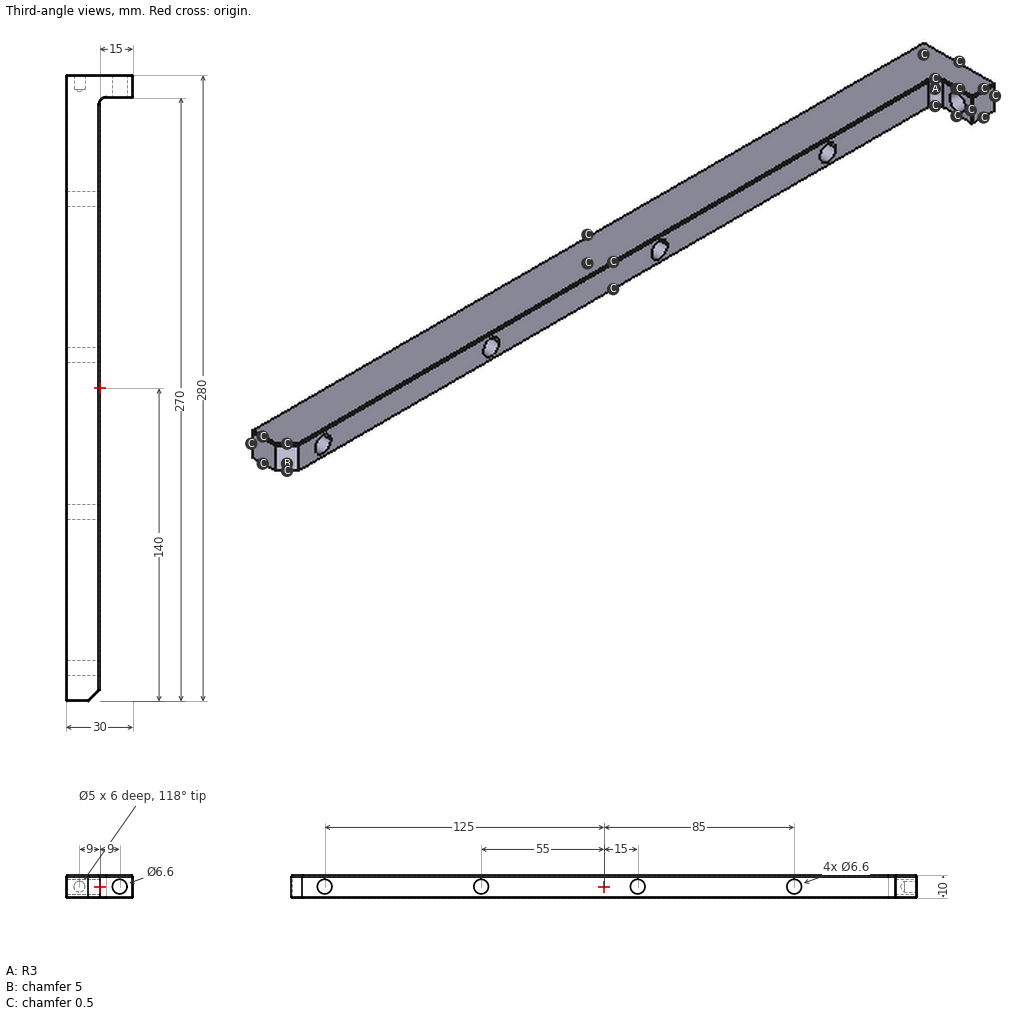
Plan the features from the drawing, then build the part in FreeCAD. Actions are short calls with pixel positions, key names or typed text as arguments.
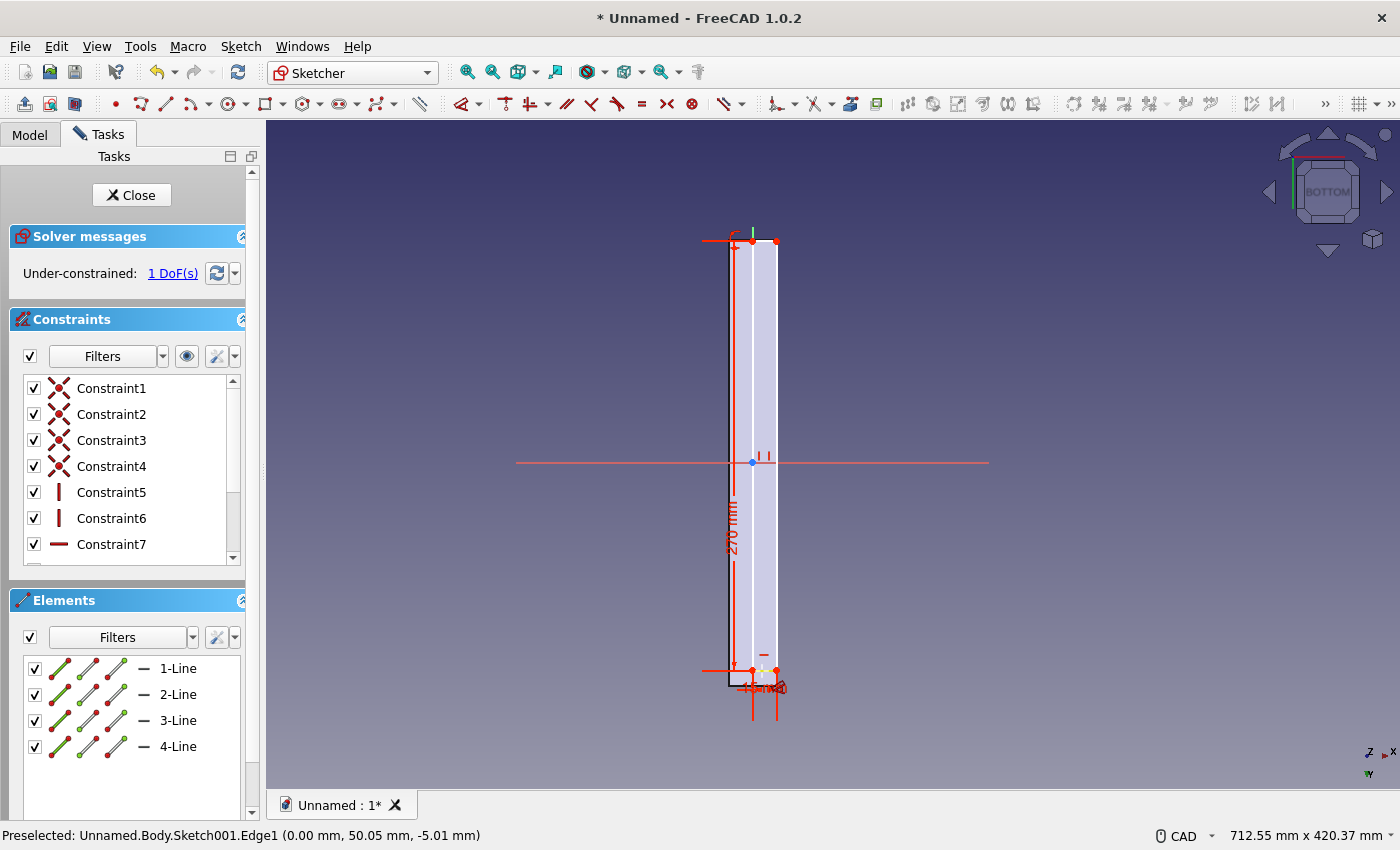
click(753, 241)
click(719, 352)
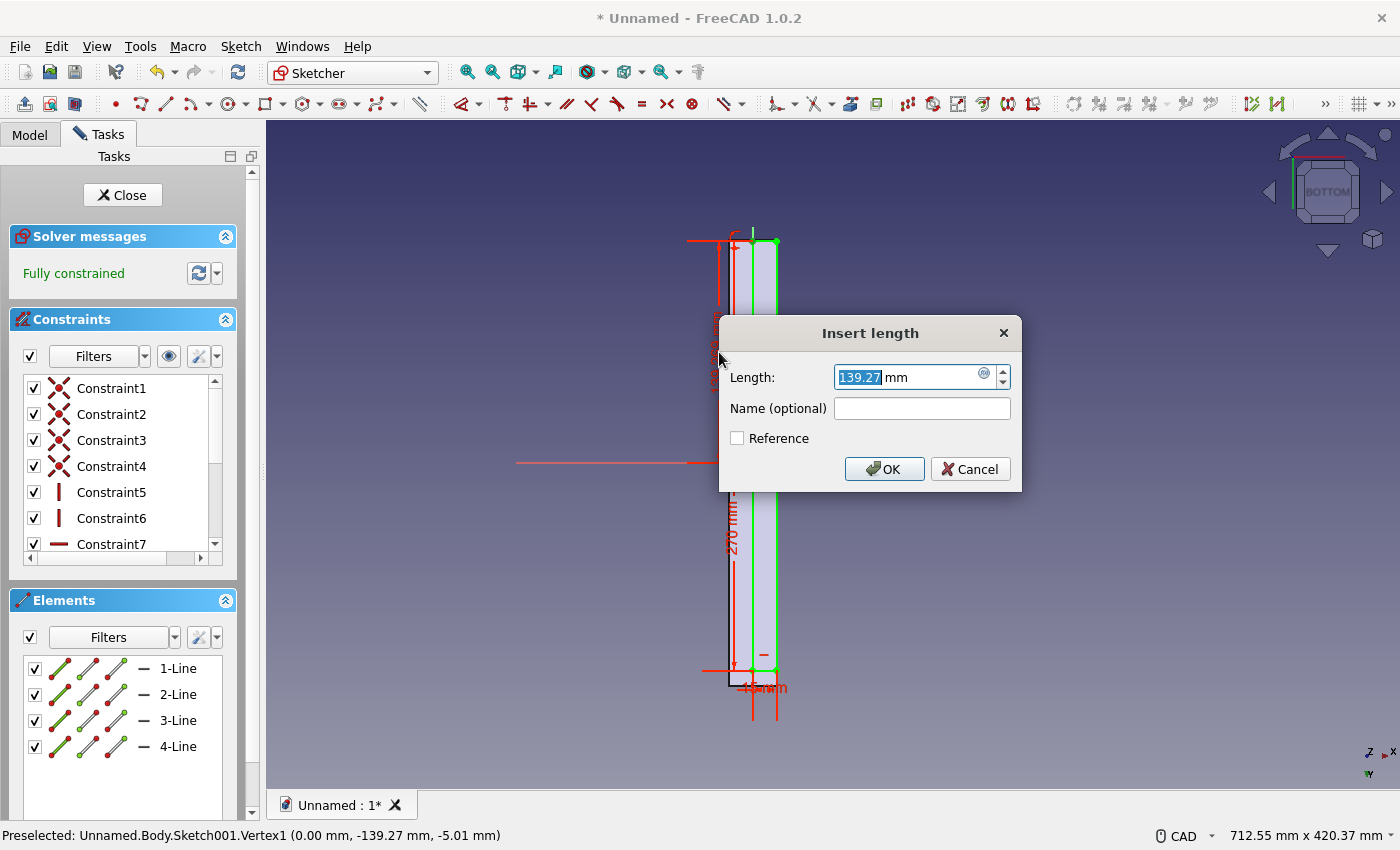
text(140)
key(Return)
key(Escape)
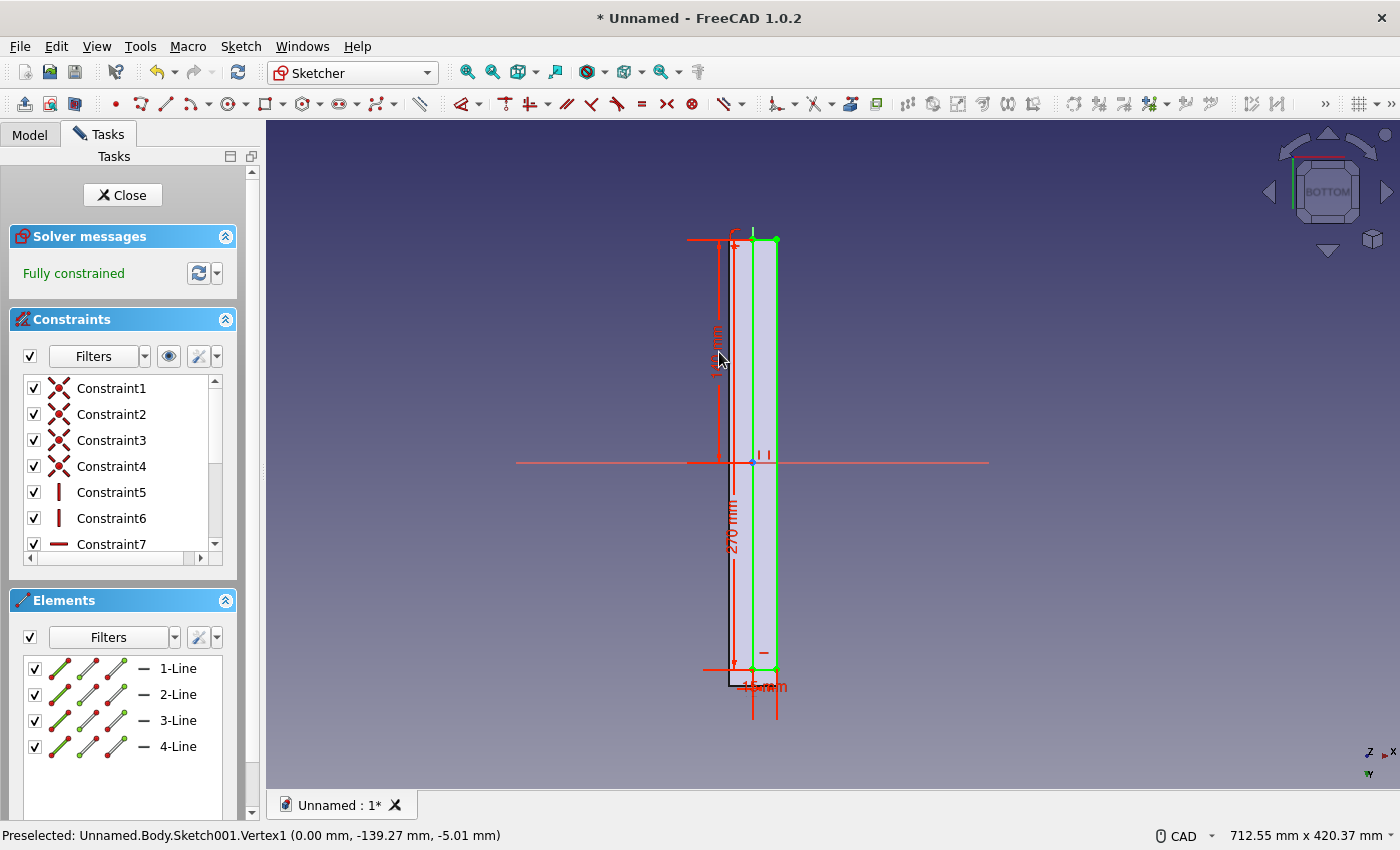
click(123, 195)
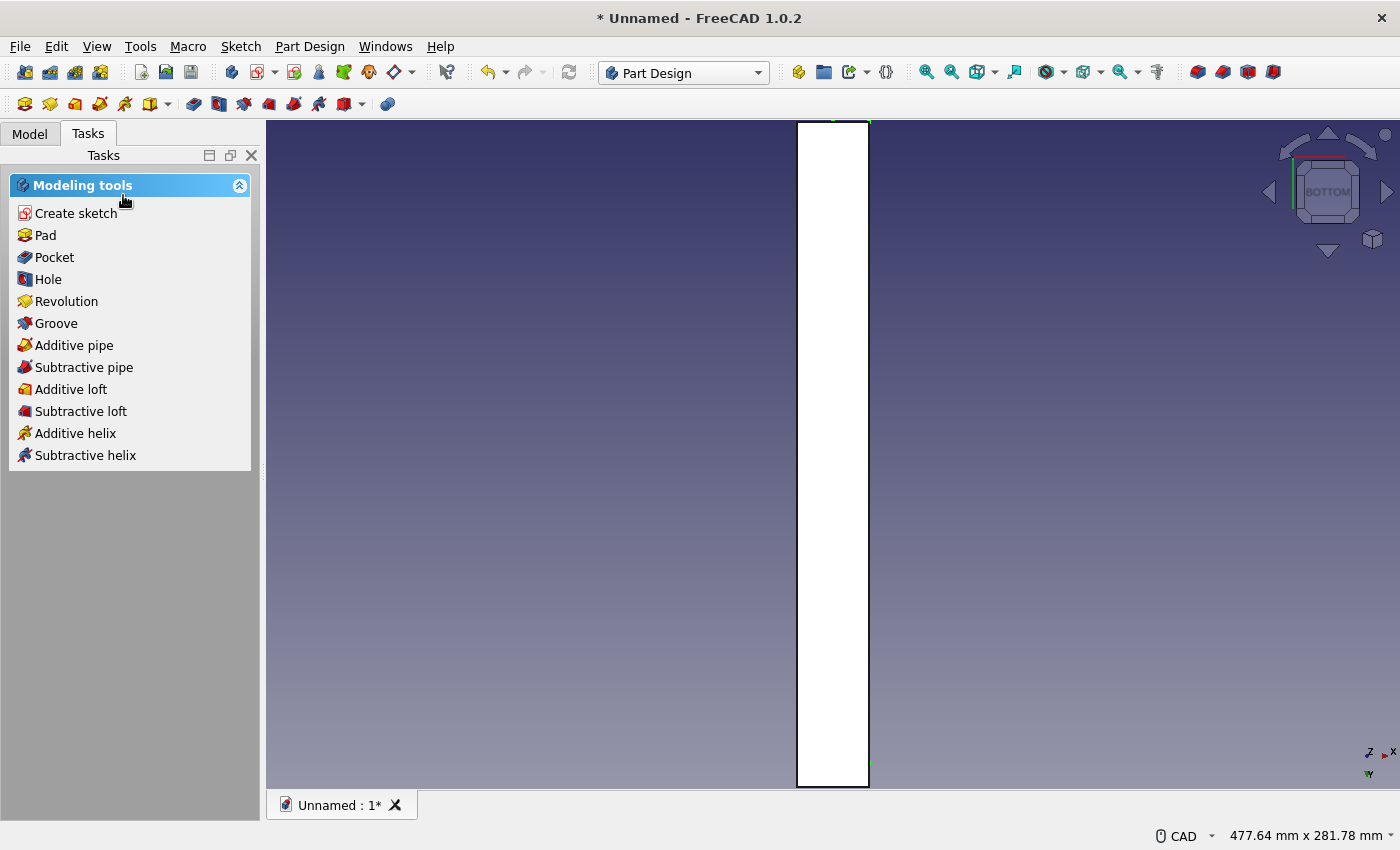
click(194, 104)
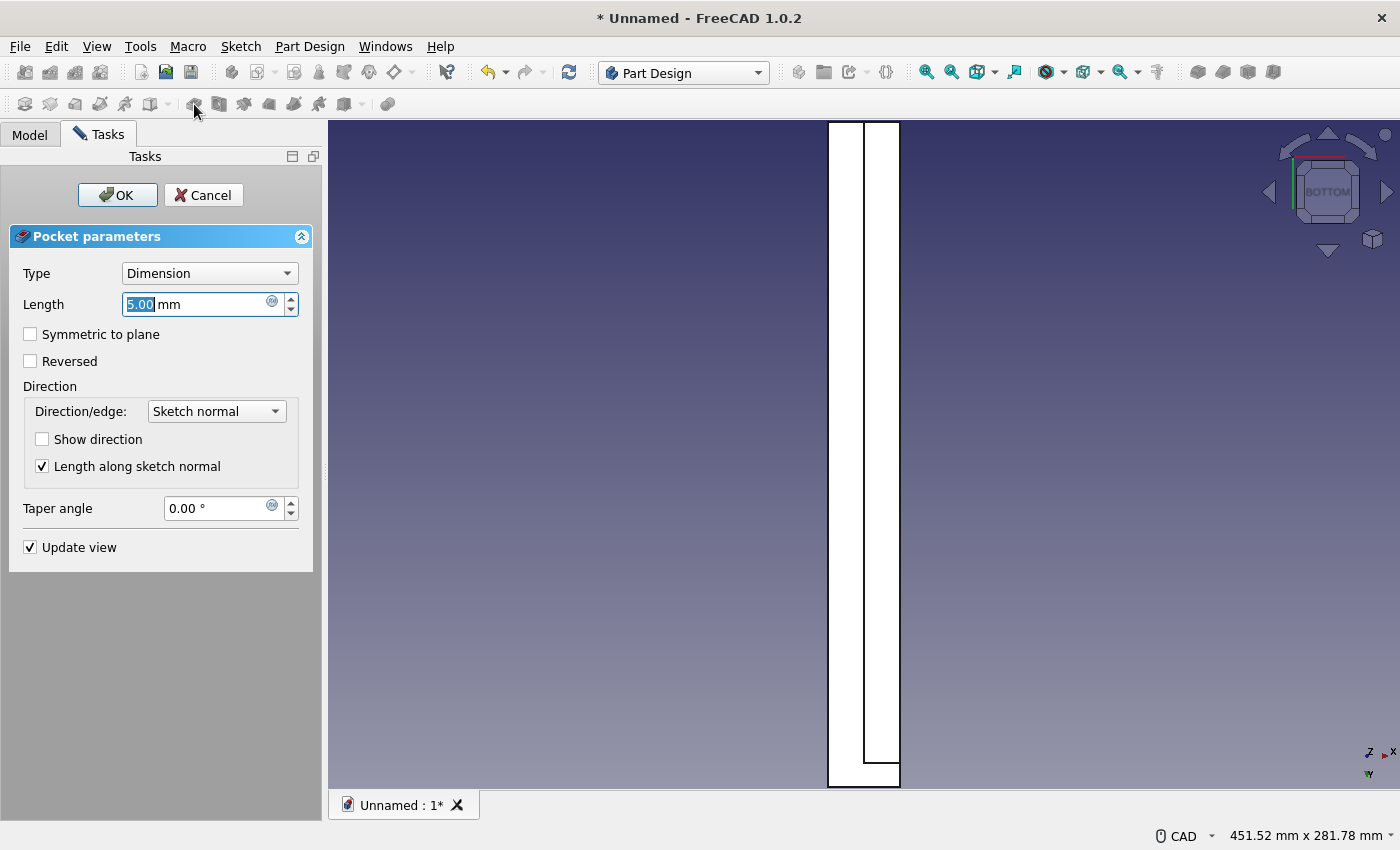
click(210, 274)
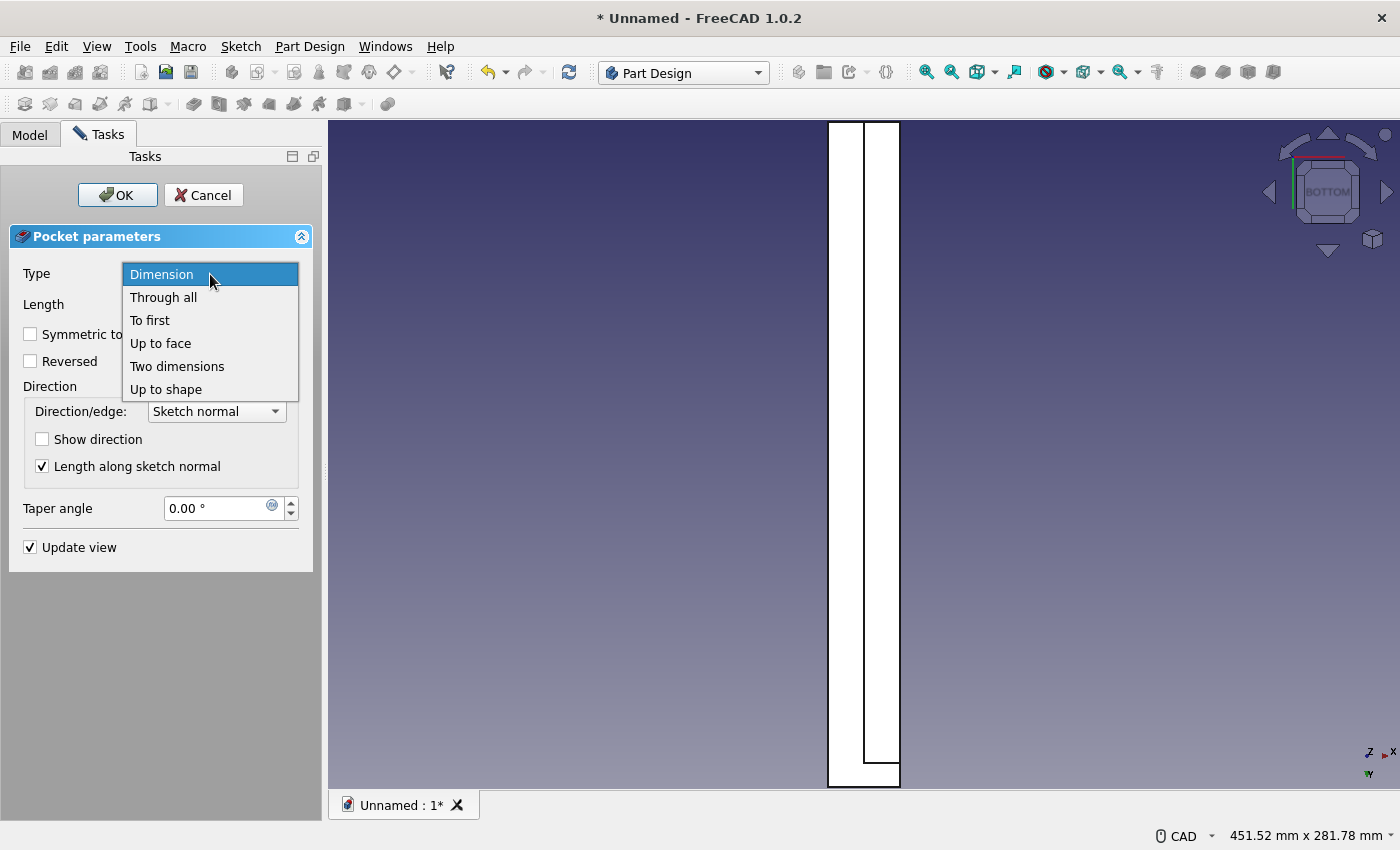
click(208, 298)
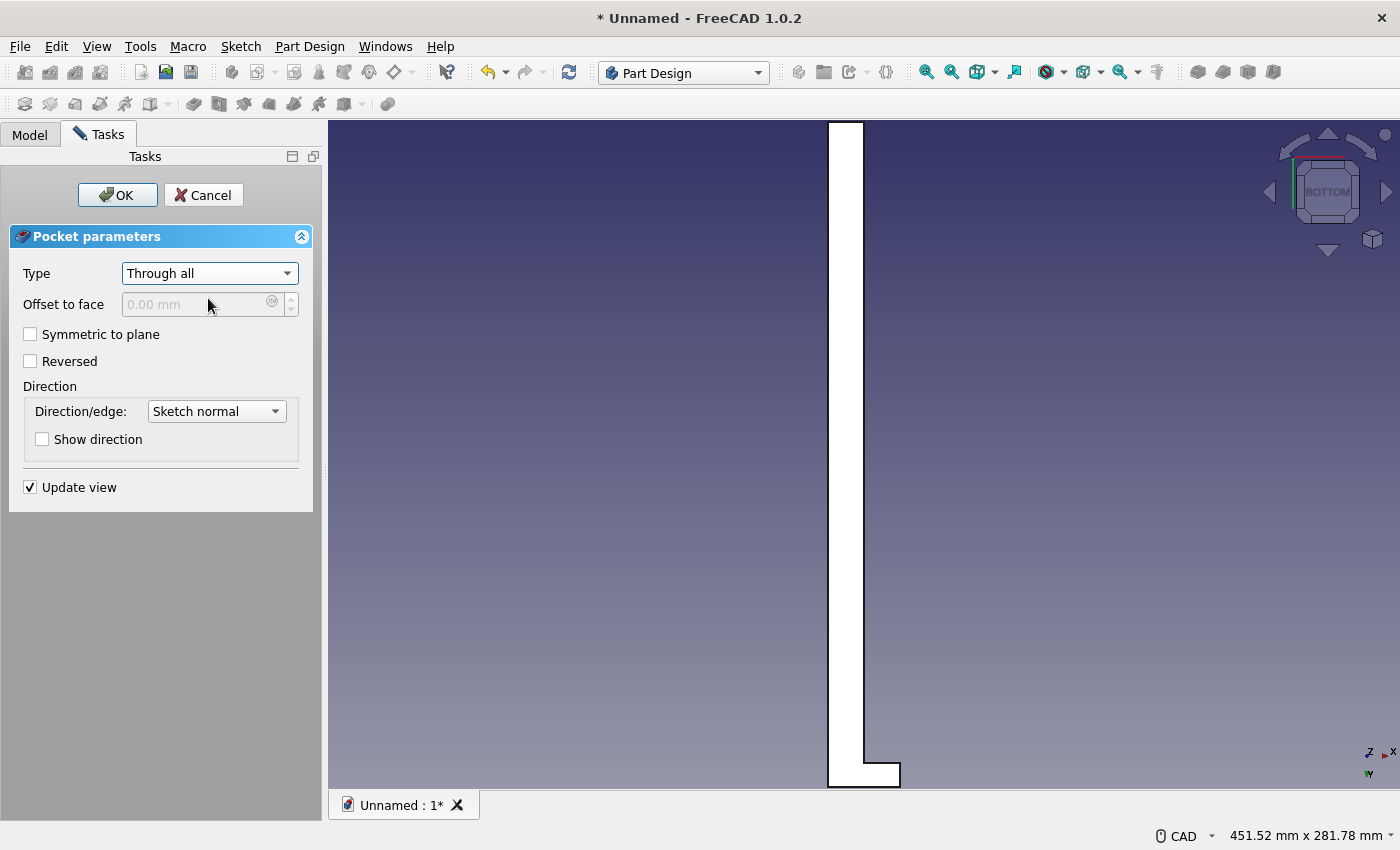
click(118, 195)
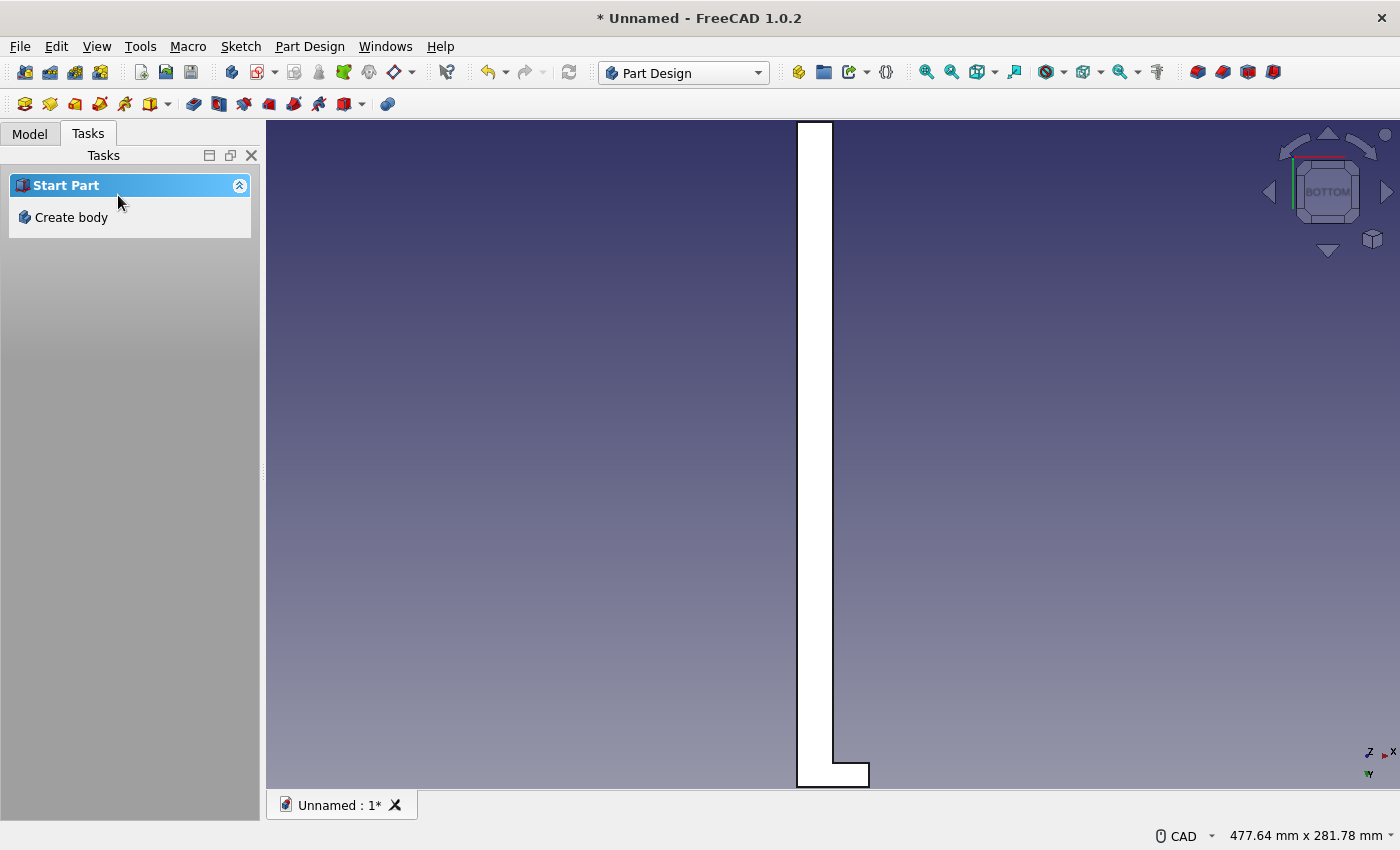
key(0)